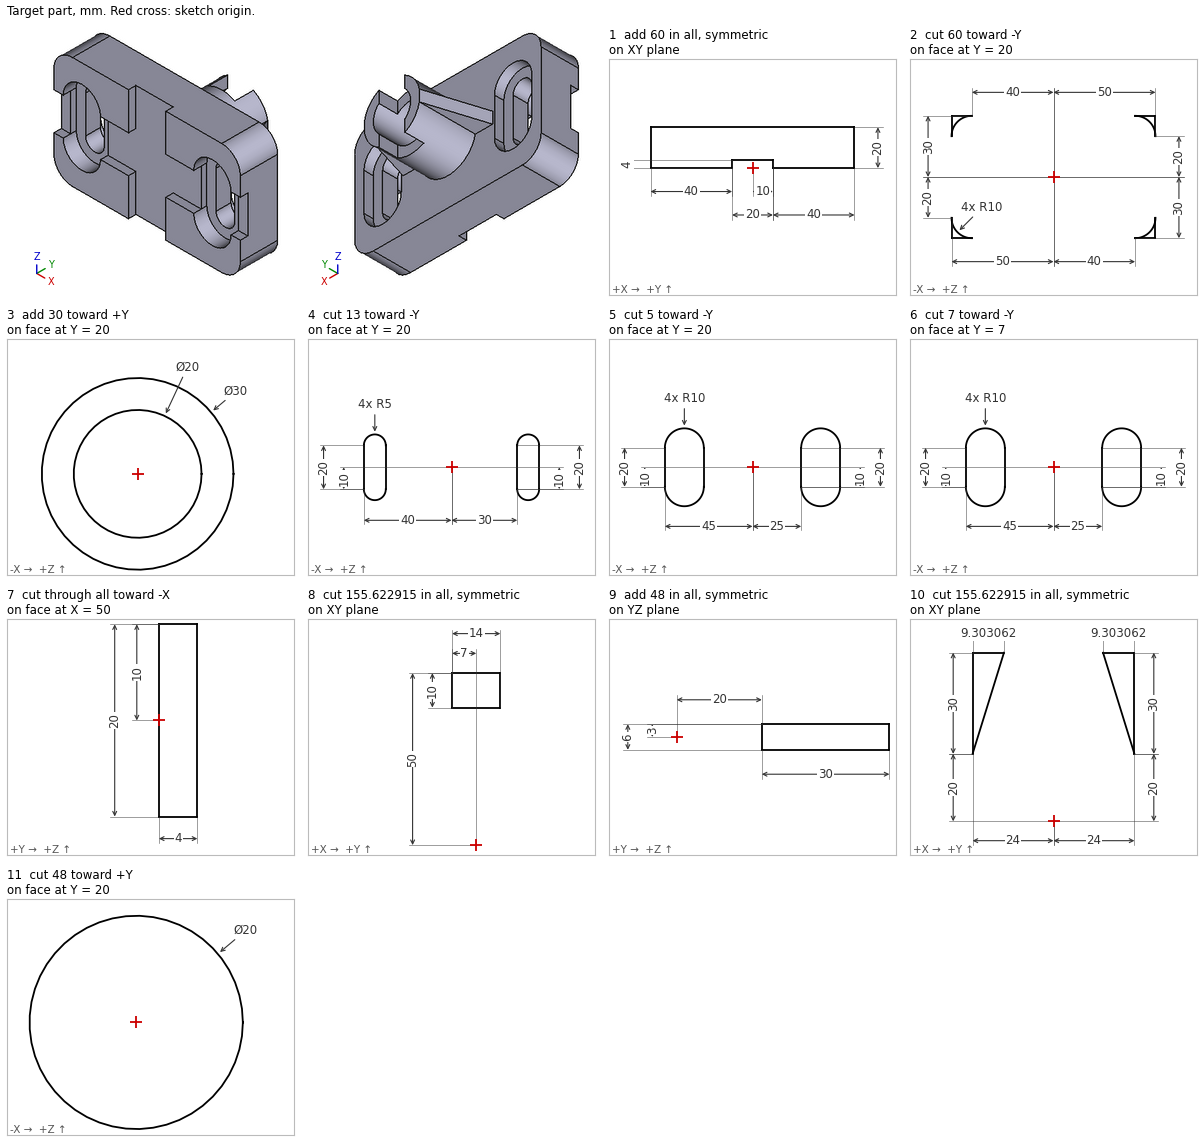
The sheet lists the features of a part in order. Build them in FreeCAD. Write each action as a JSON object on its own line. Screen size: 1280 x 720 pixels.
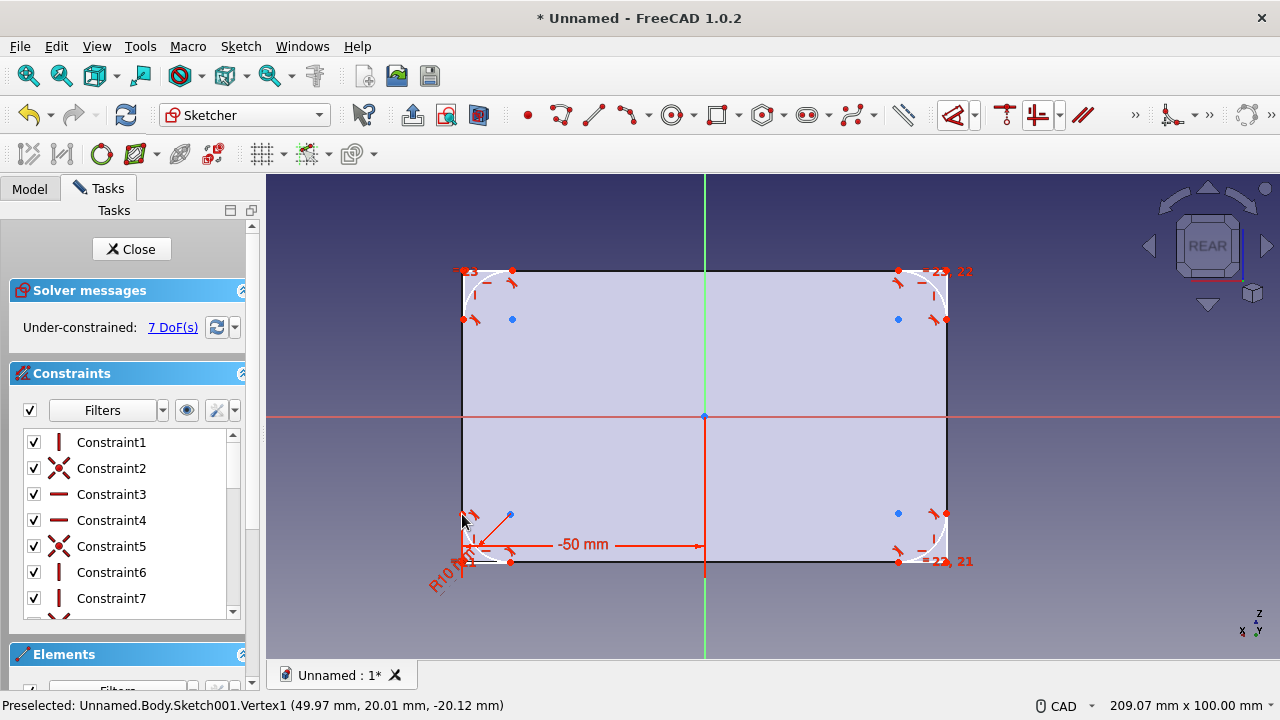
{"action": "left_click", "coordinate": [462, 514]}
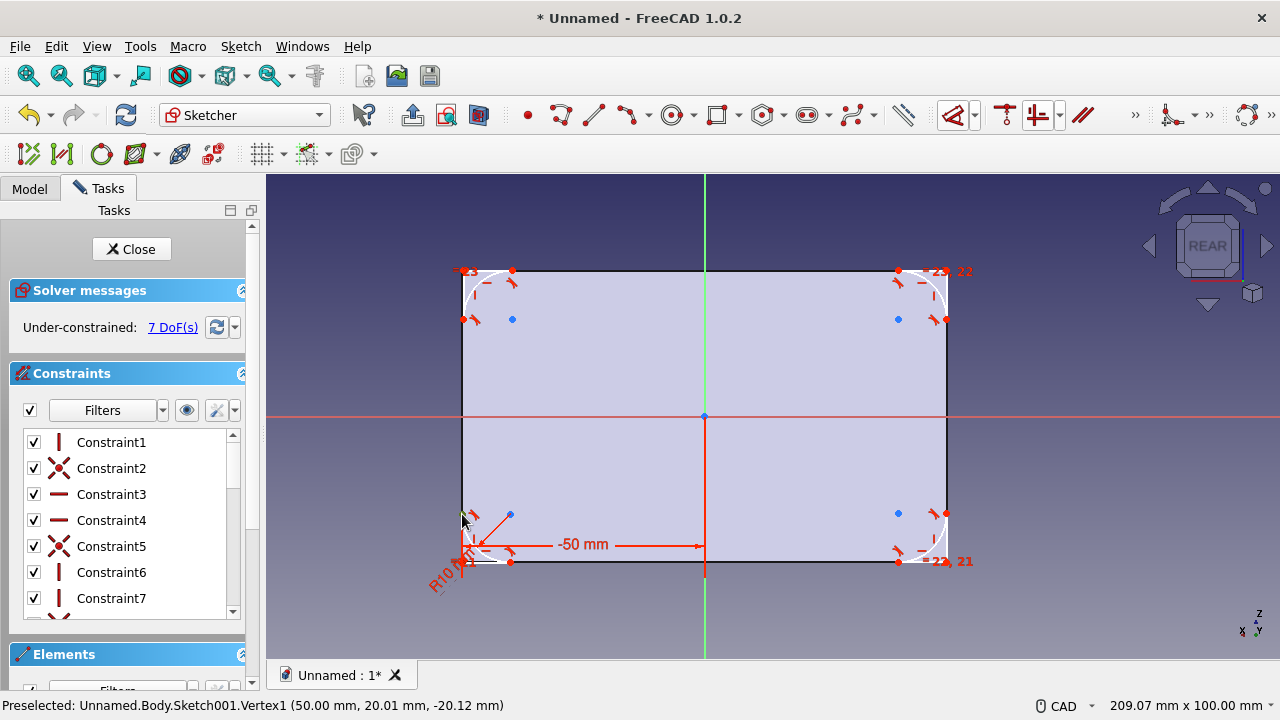
{"action": "key", "text": "i"}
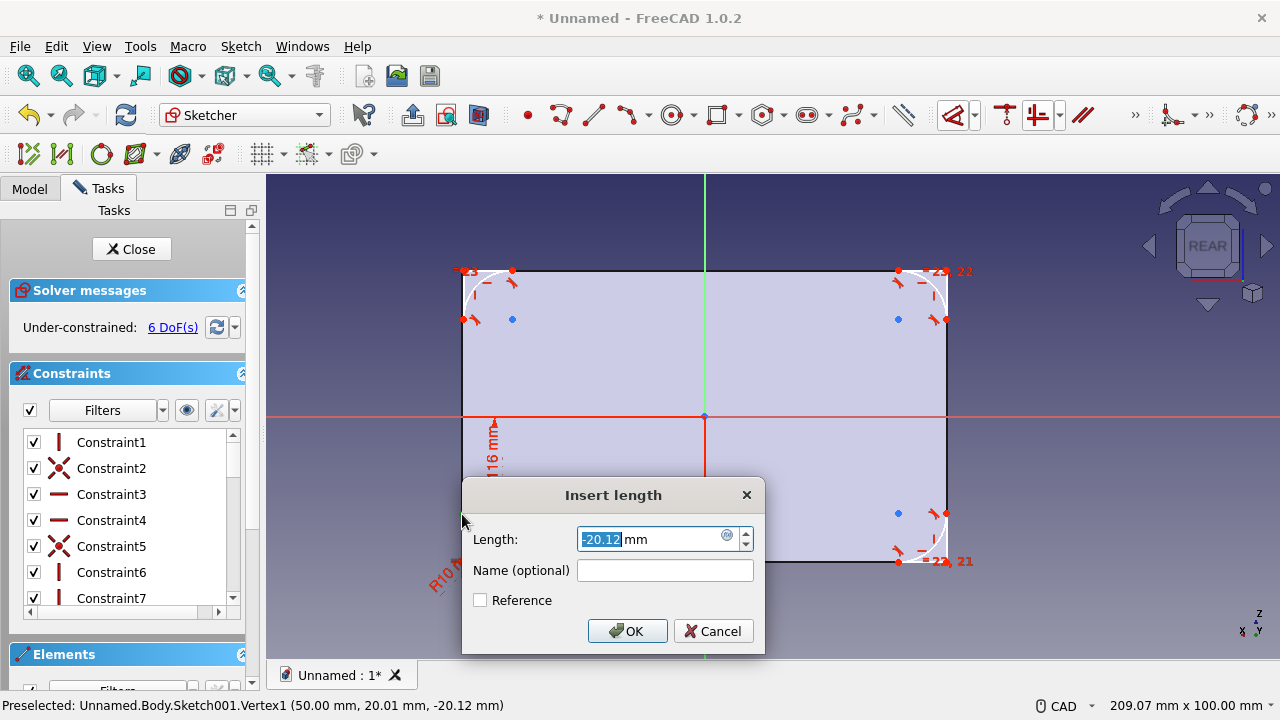
{"action": "type", "text": "-20"}
{"action": "key", "text": "Return"}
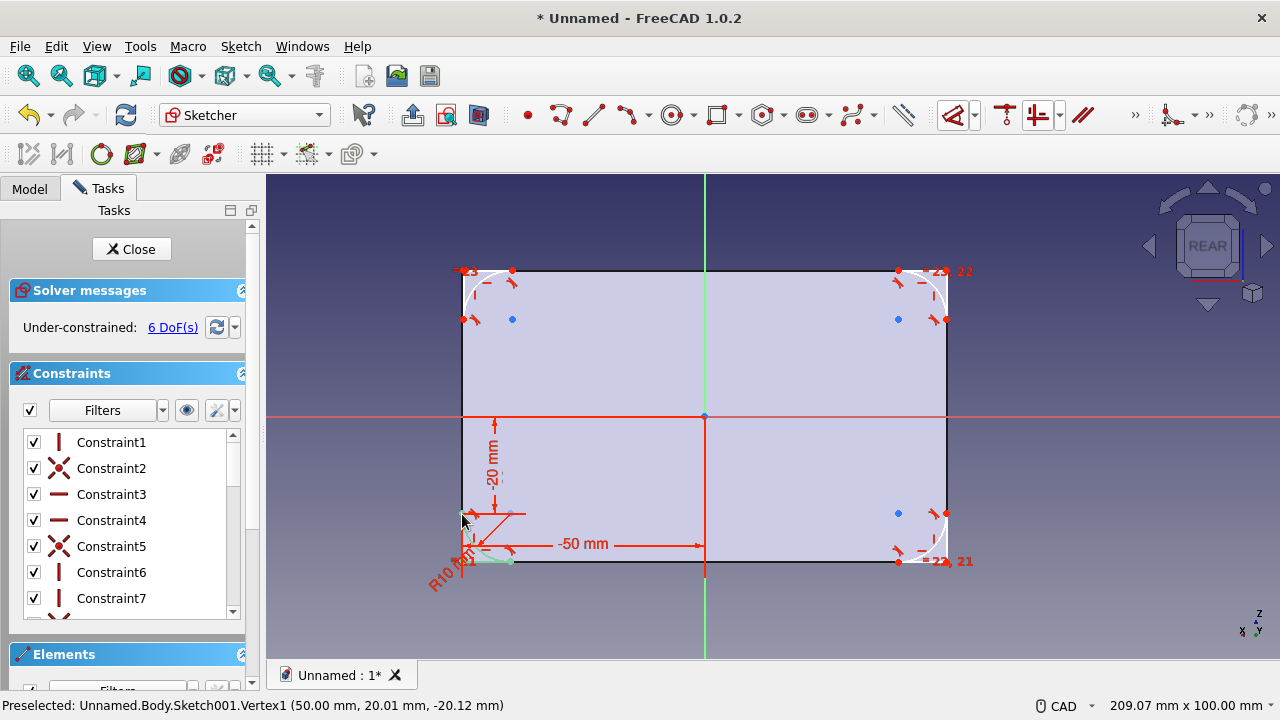
{"action": "left_click", "coordinate": [898, 562]}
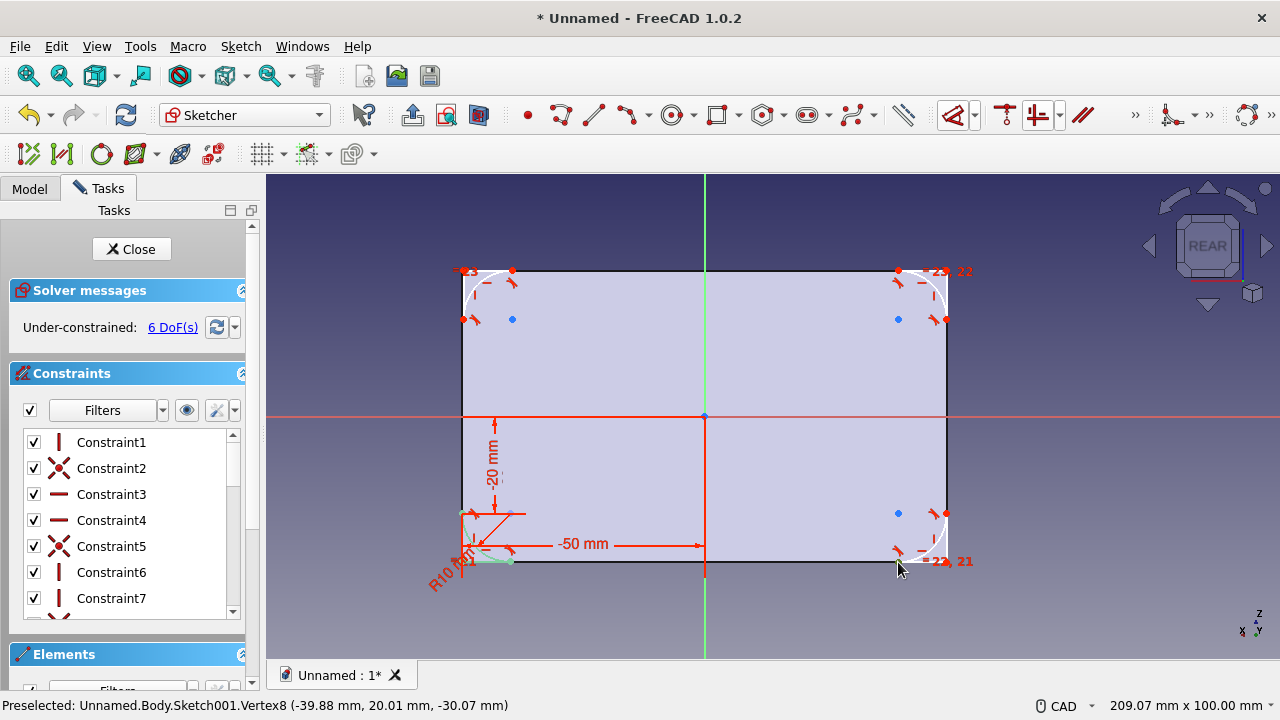
{"action": "key", "text": "l"}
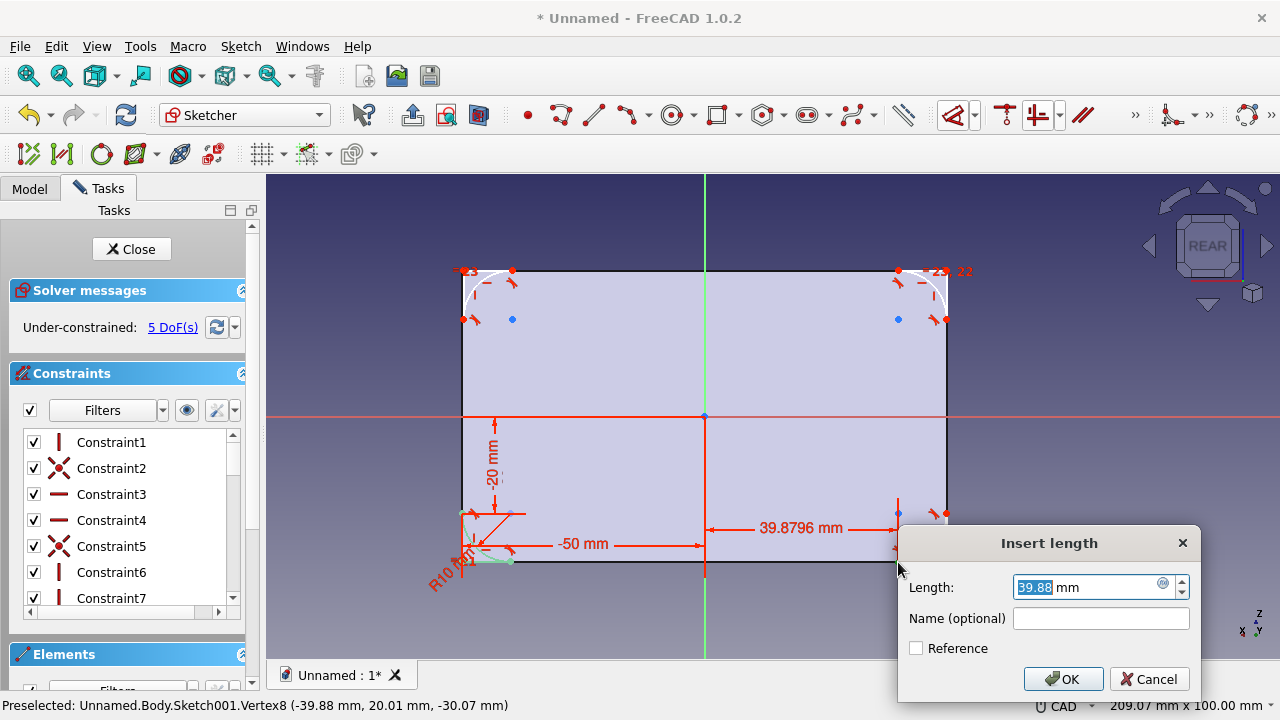
{"action": "type", "text": "40"}
{"action": "key", "text": "Return"}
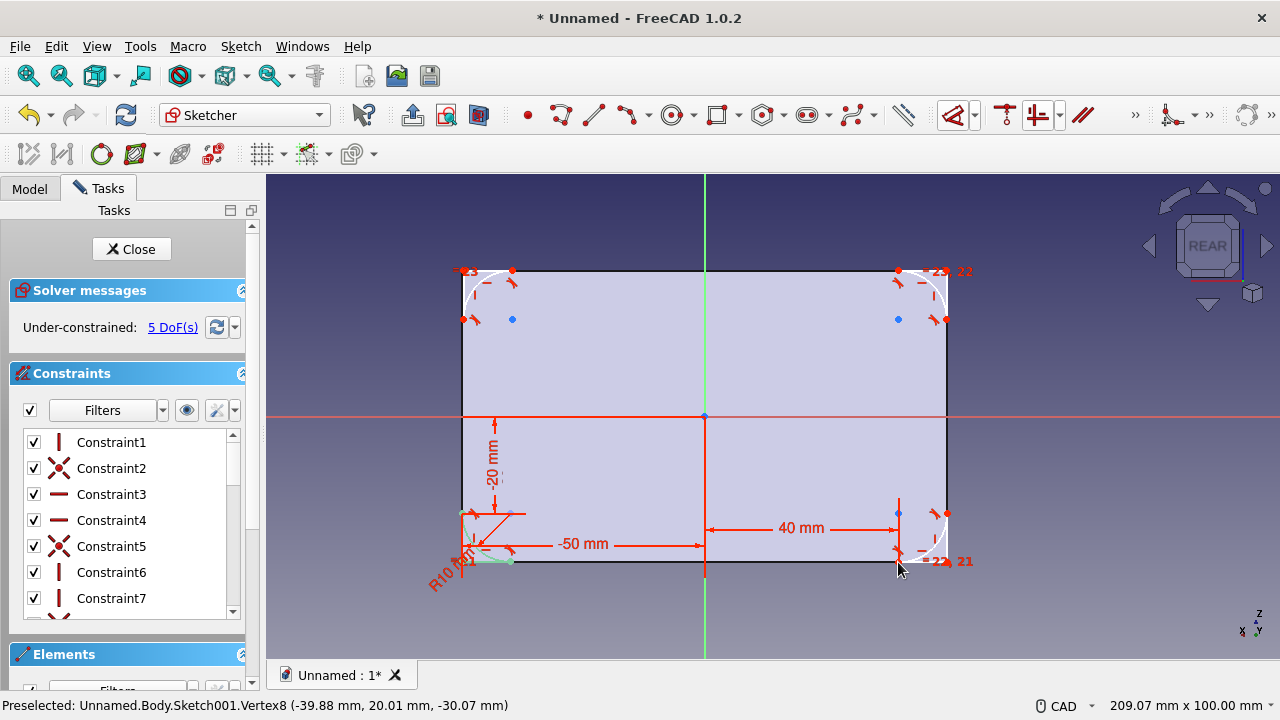
{"action": "left_click", "coordinate": [899, 562]}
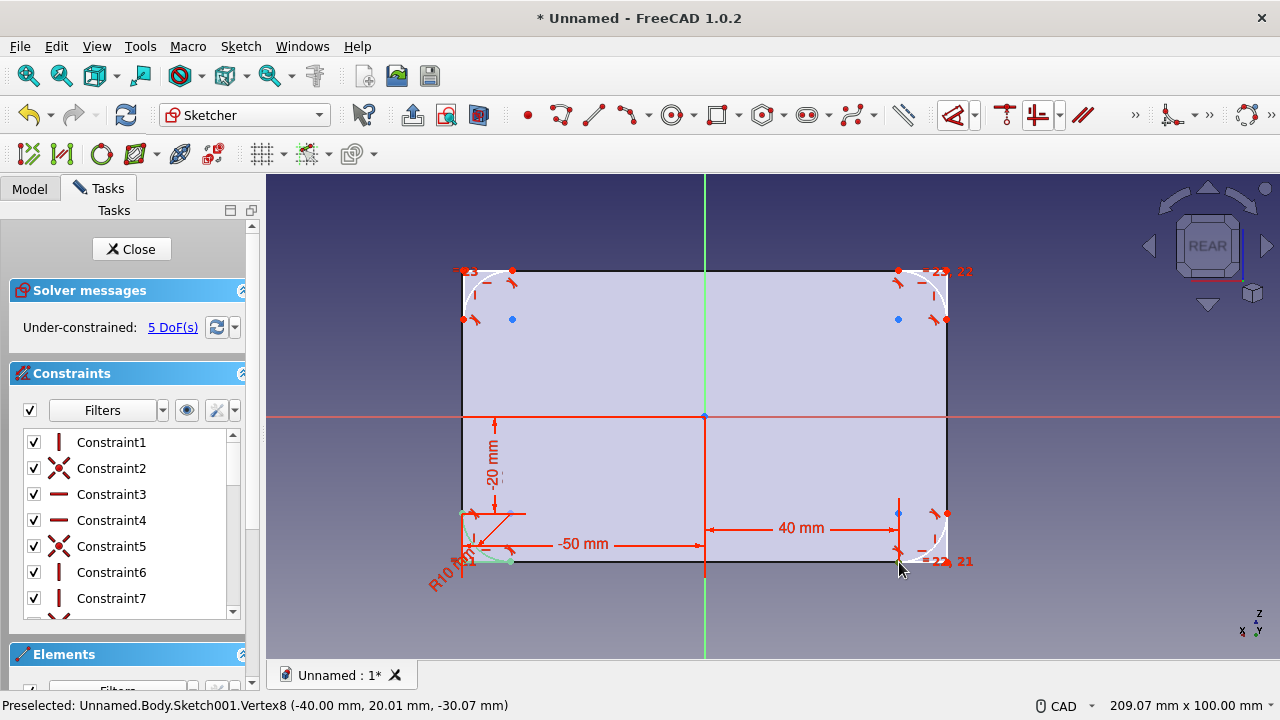
{"action": "key", "text": "i"}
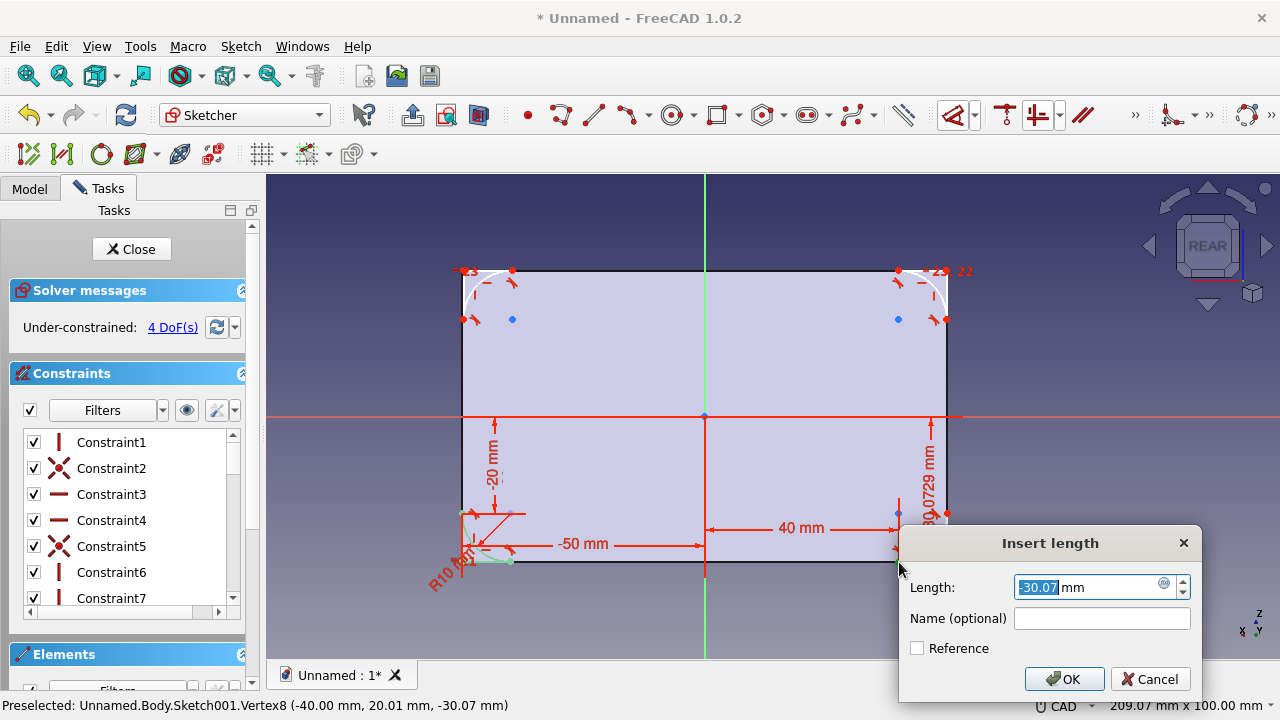
{"action": "type", "text": "-30"}
{"action": "key", "text": "Return"}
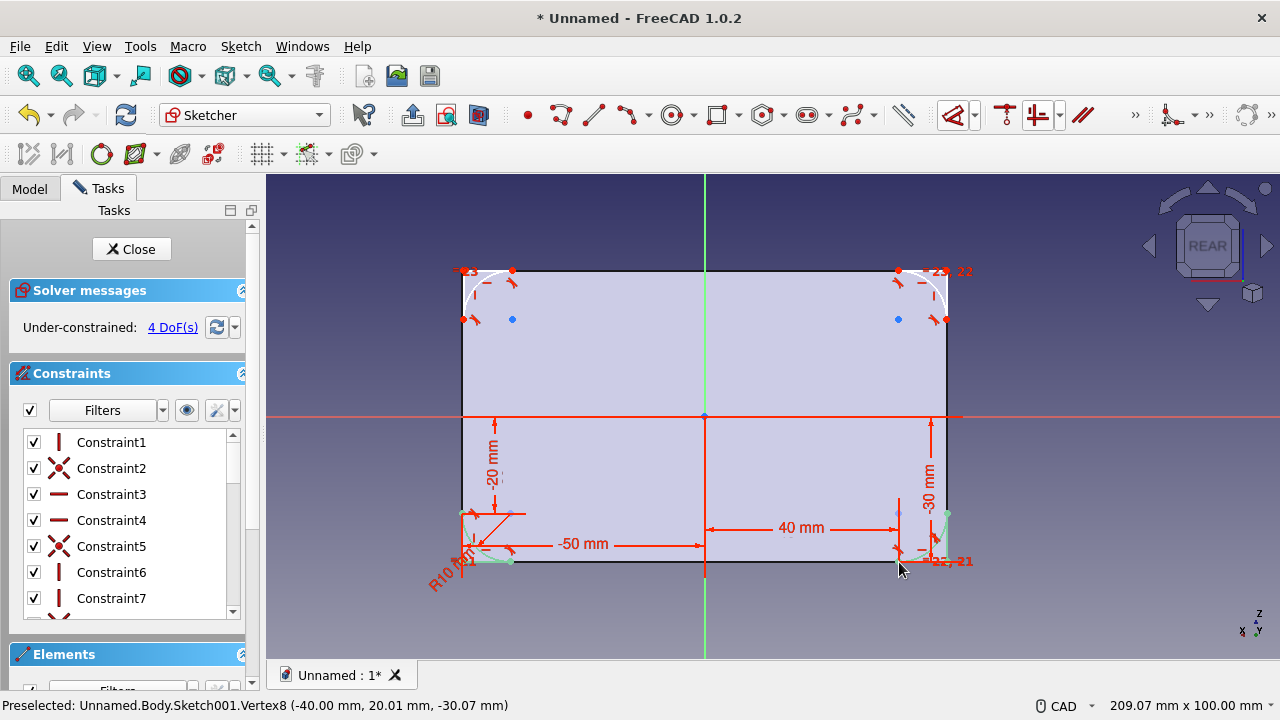
{"action": "left_click", "coordinate": [947, 319]}